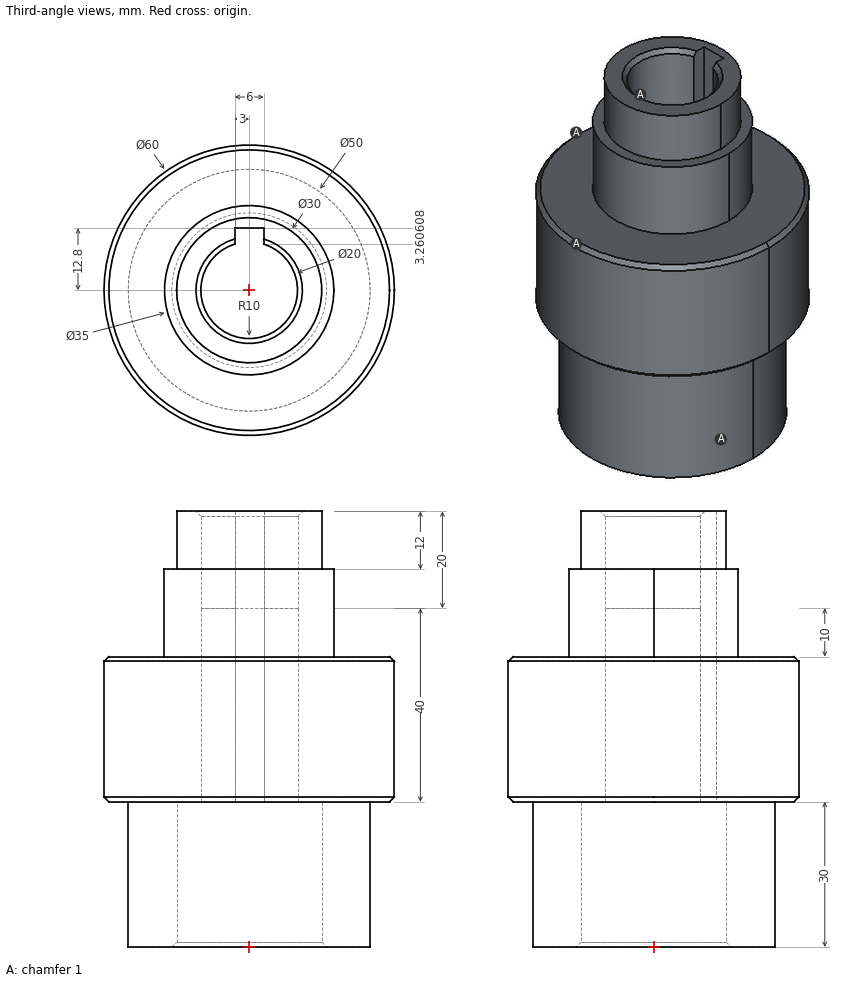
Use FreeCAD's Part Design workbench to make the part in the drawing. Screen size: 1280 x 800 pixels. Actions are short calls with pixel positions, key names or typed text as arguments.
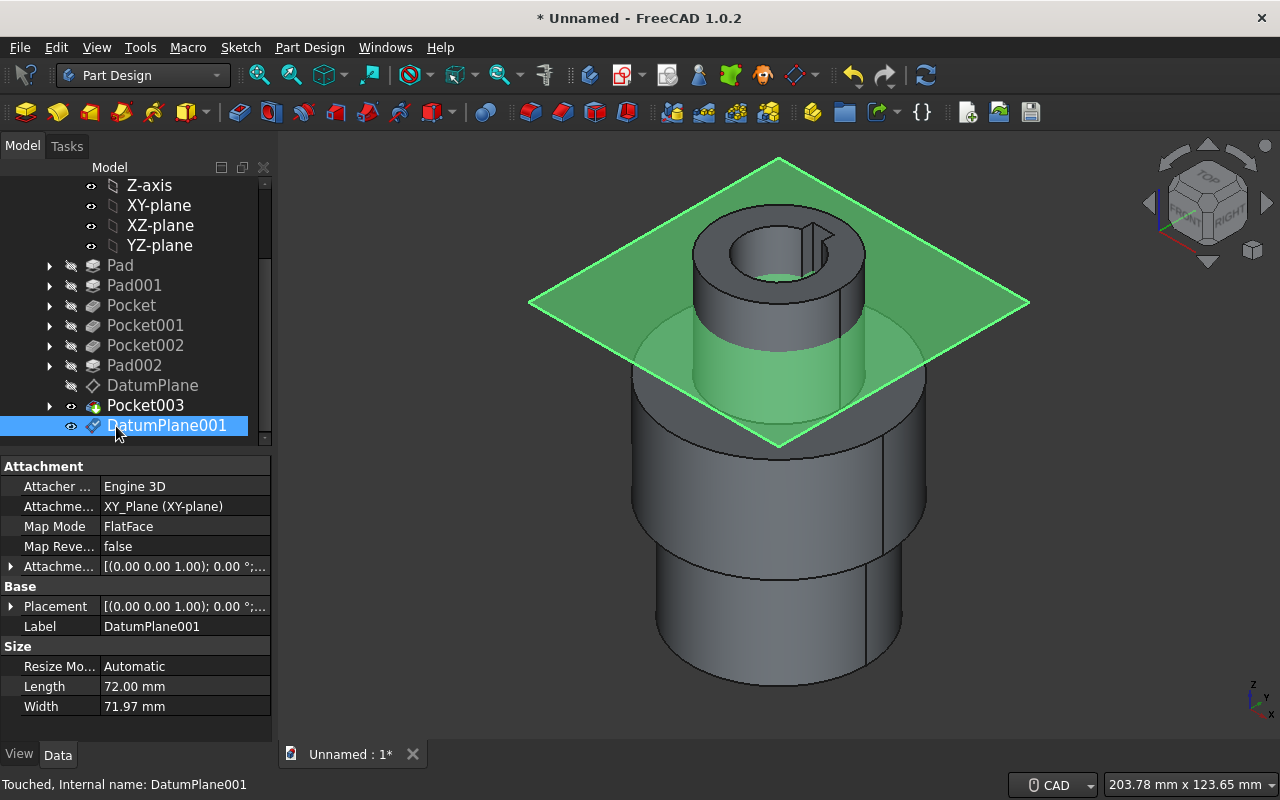
click(622, 76)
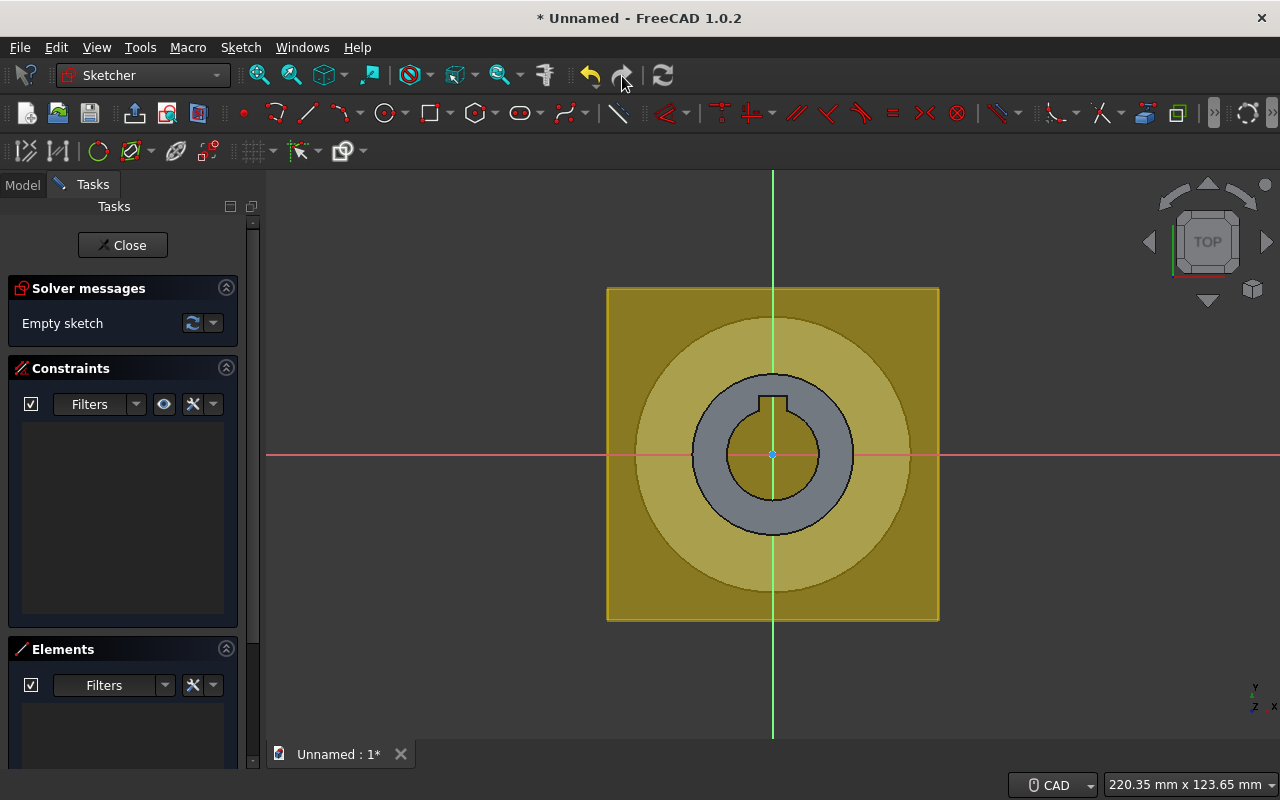
click(200, 114)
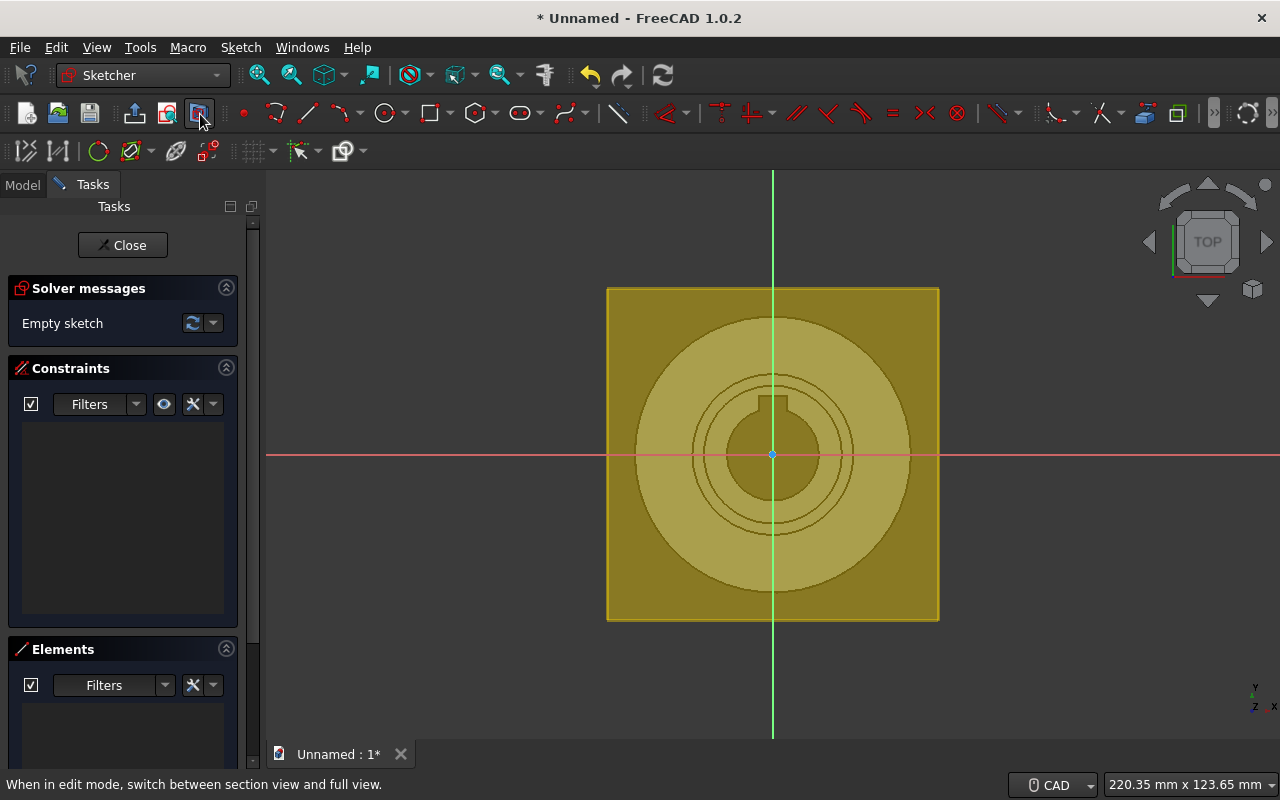
scroll(829, 455, up, 4)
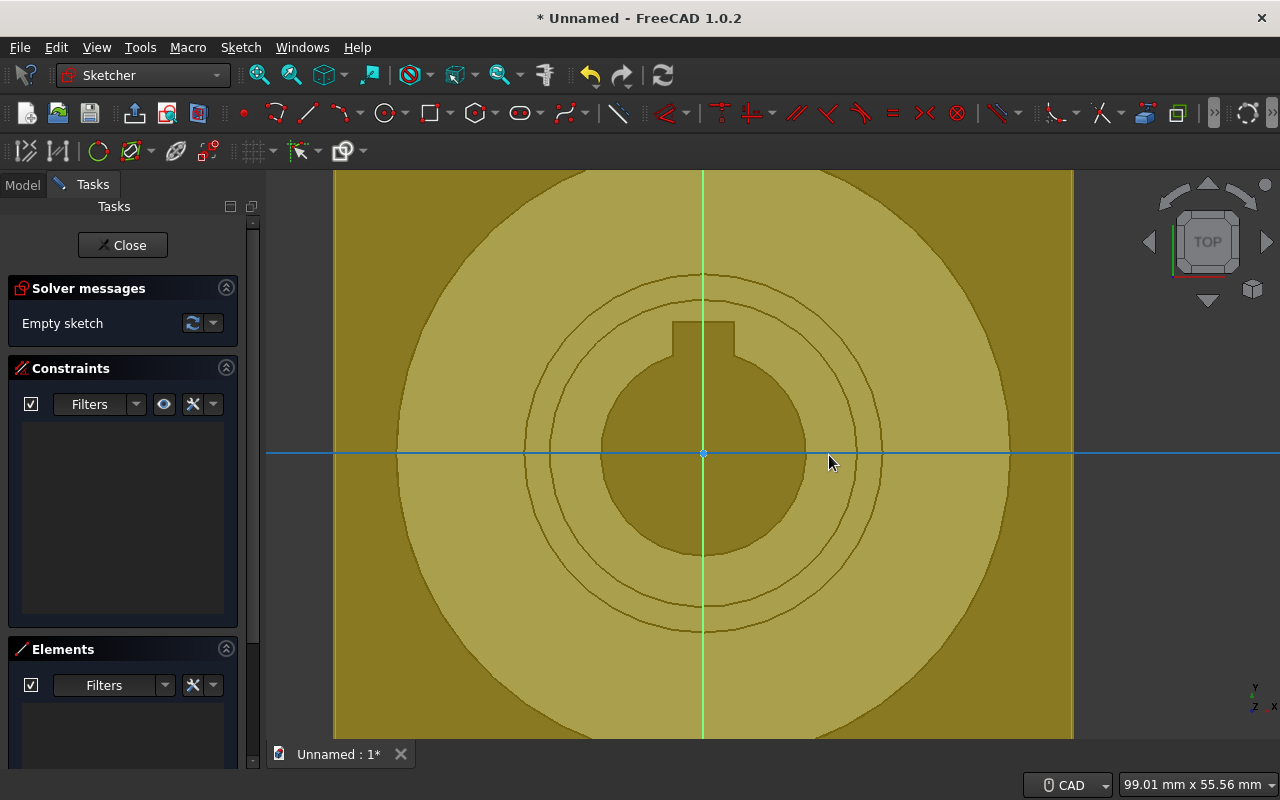
key(g)
key(c)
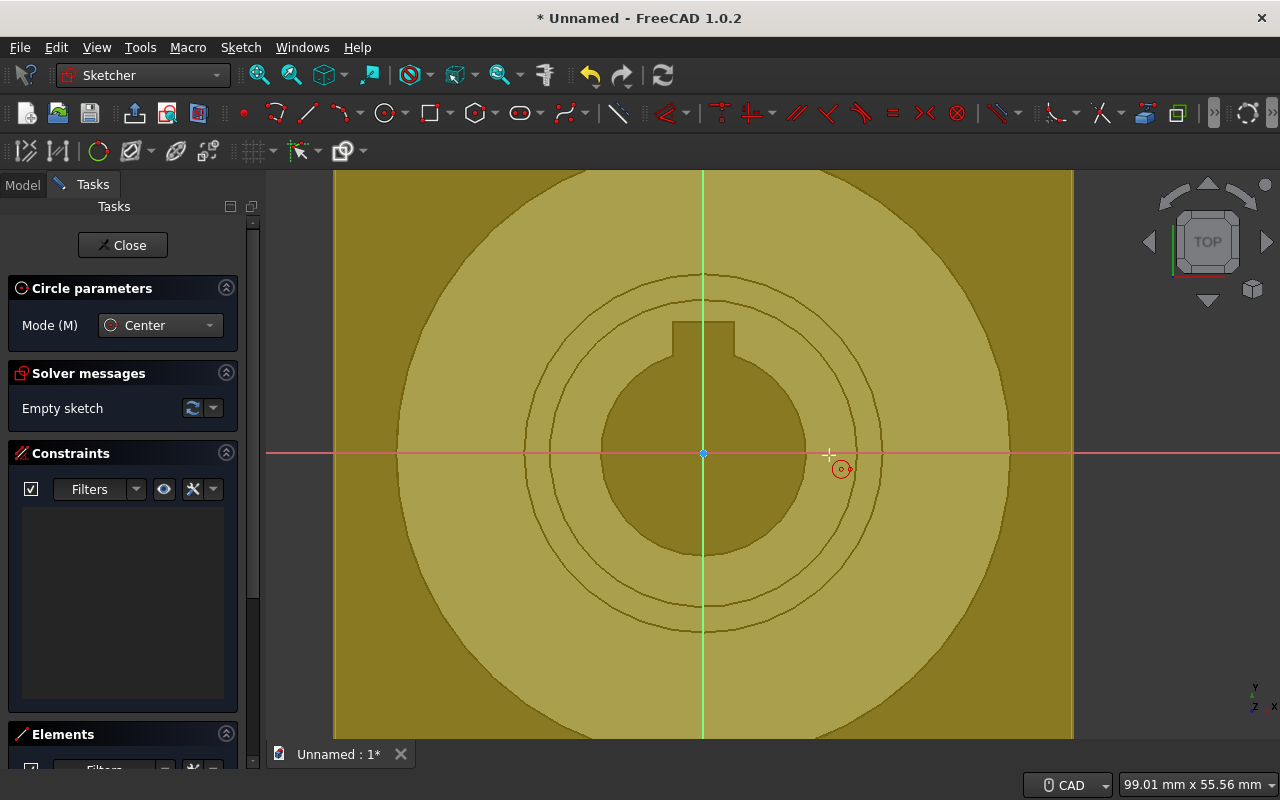
click(703, 453)
move(830, 327)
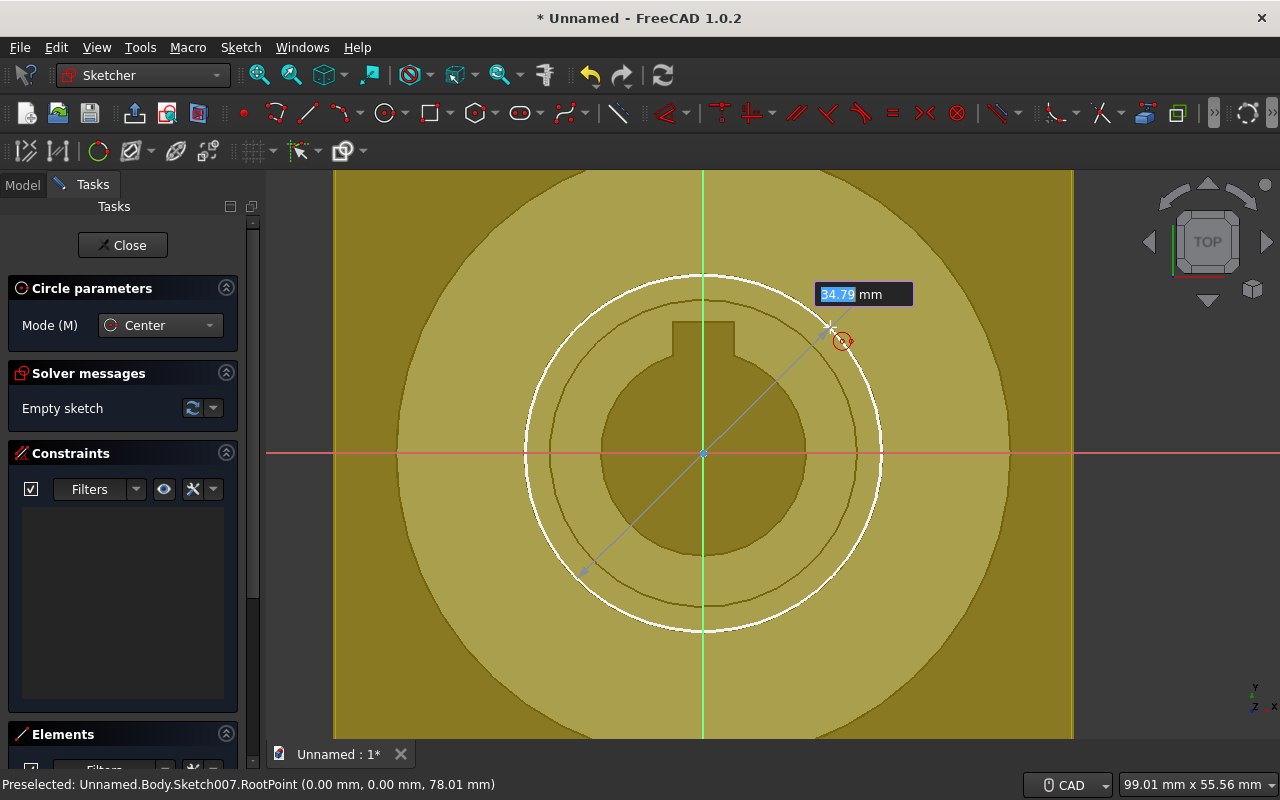
text(35)
key(Return)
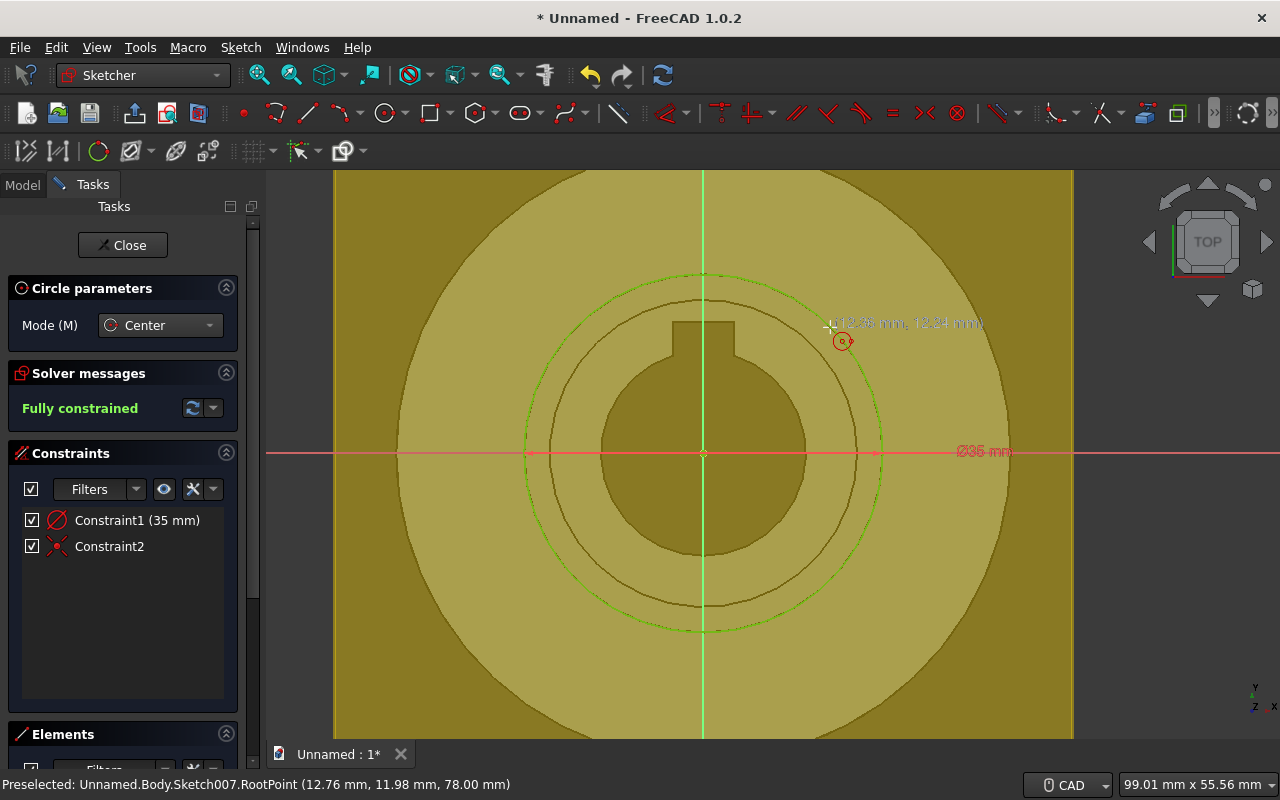
click(703, 453)
move(812, 345)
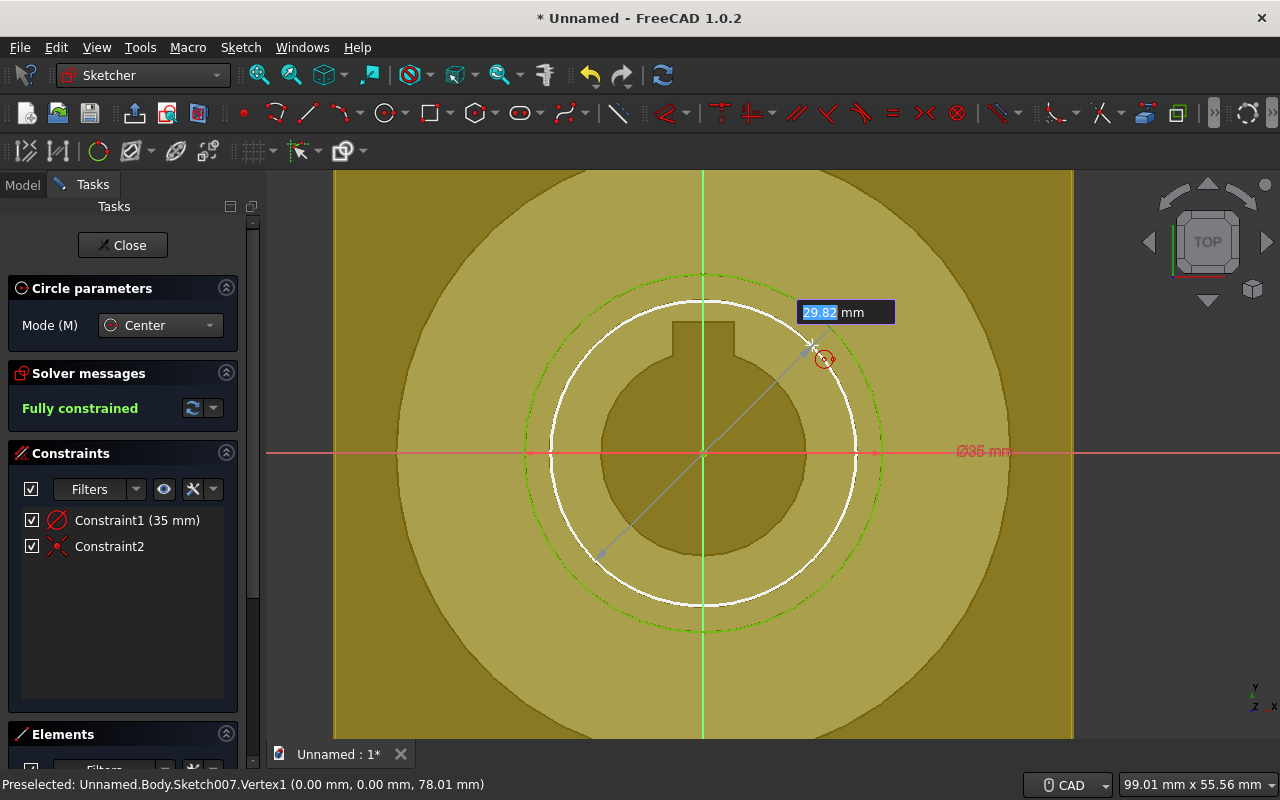
text(30)
key(Return)
key(Escape)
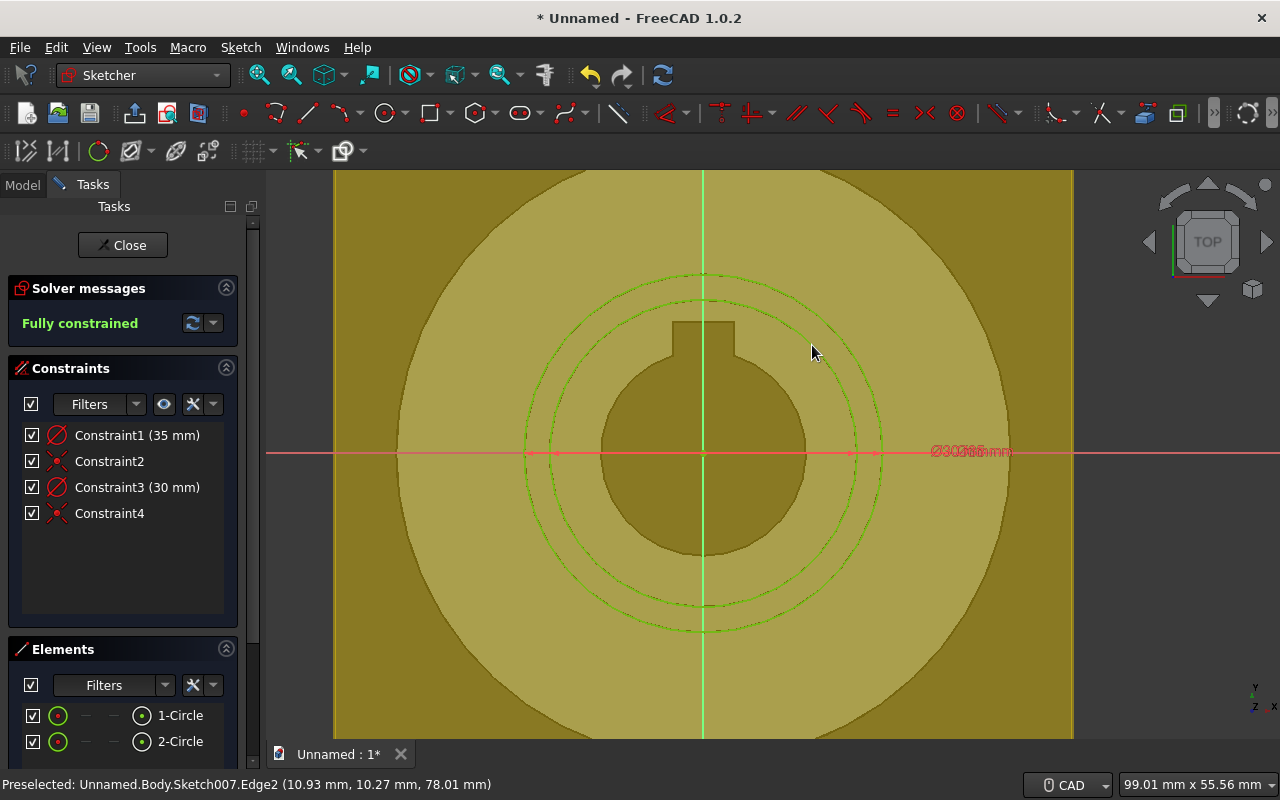
click(123, 245)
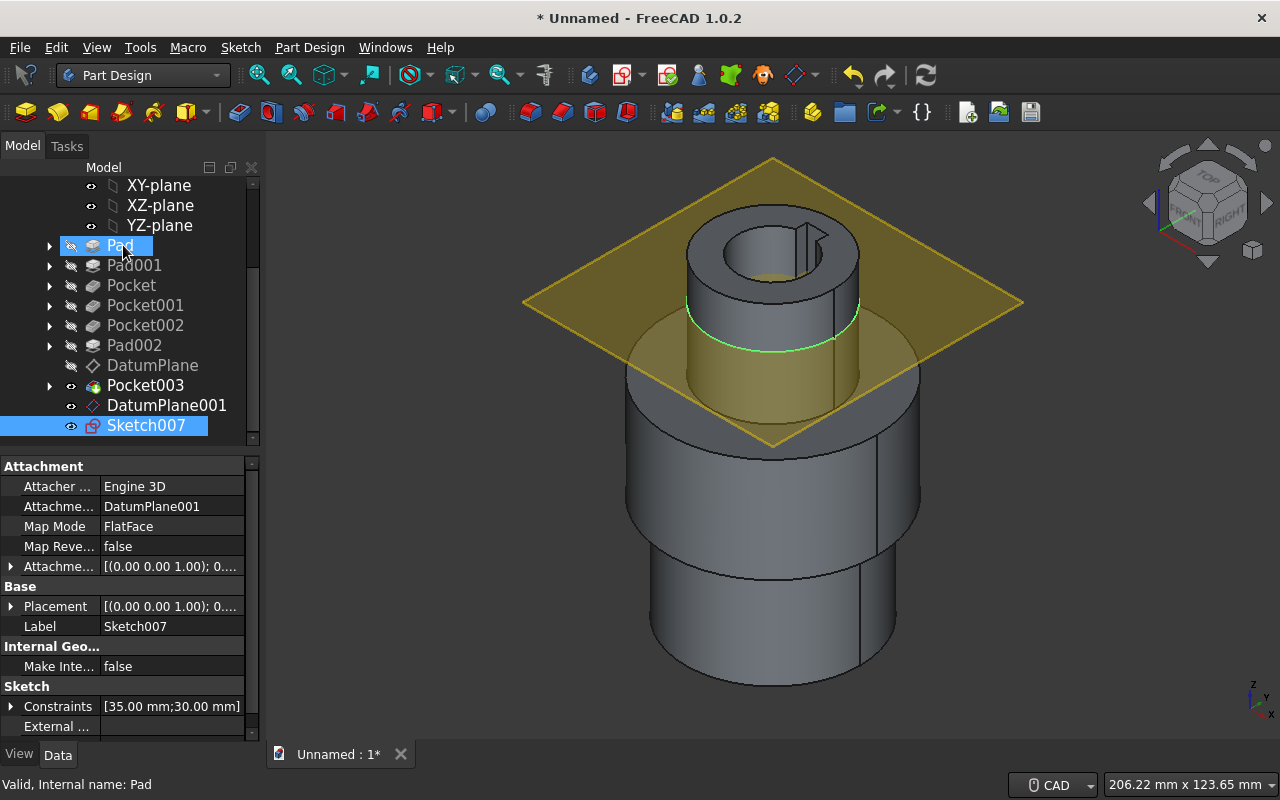
click(240, 112)